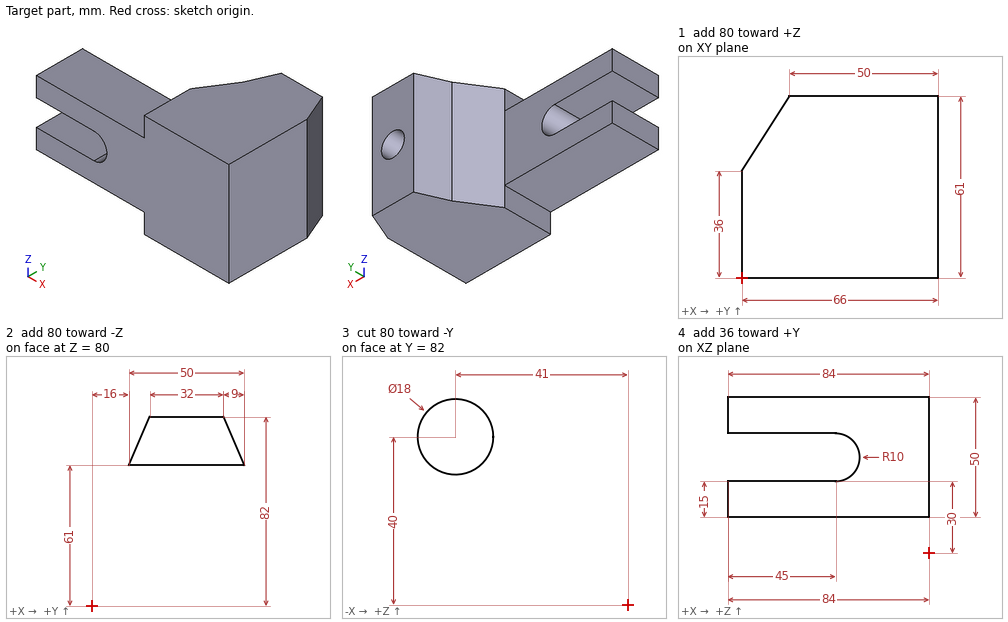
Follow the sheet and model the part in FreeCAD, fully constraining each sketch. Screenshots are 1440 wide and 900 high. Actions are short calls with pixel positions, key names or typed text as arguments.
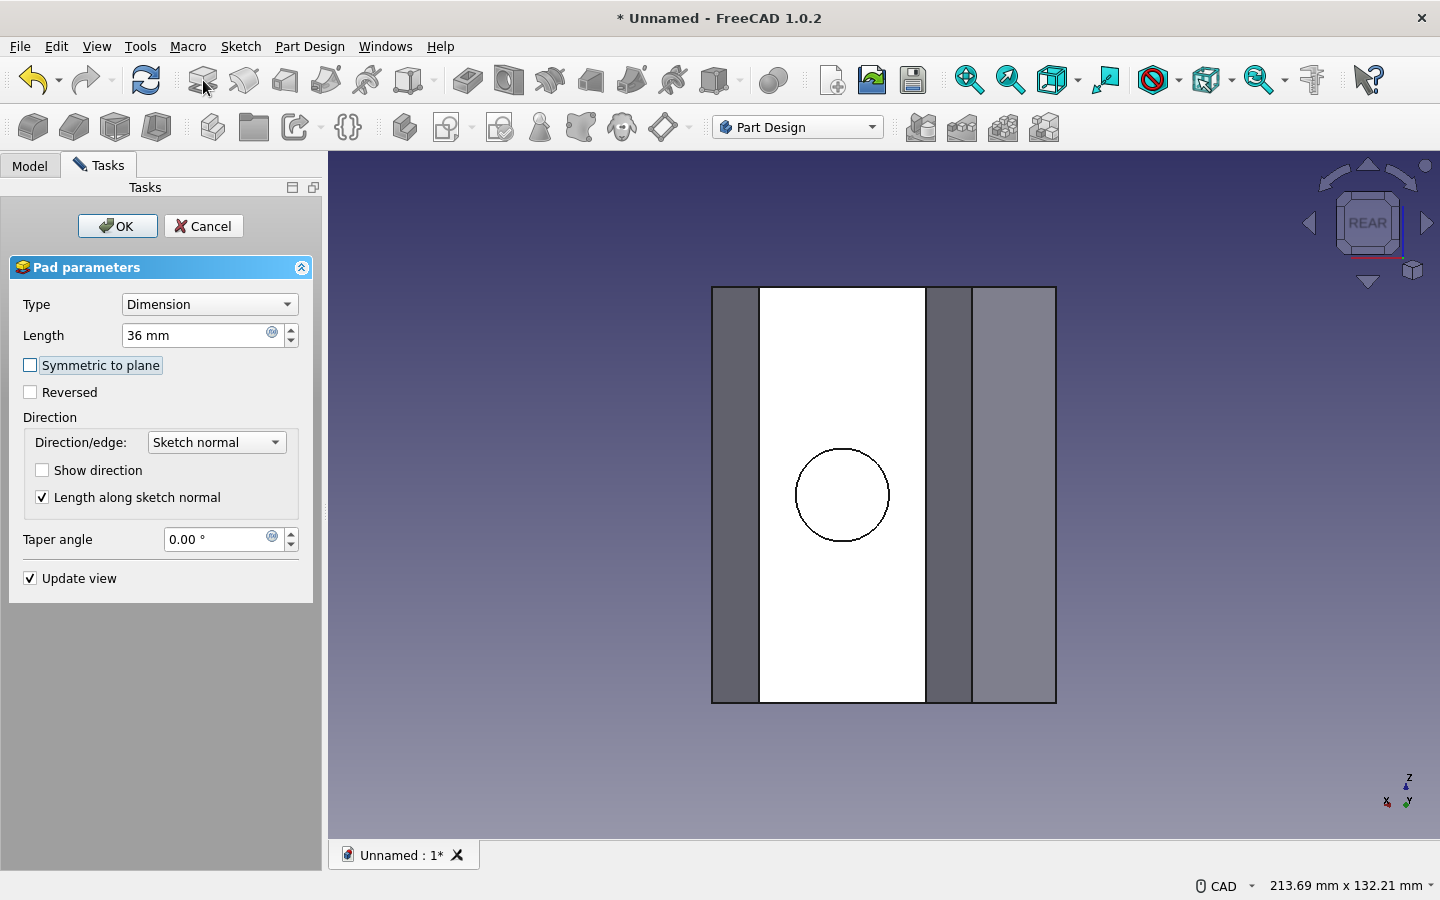
click(31, 392)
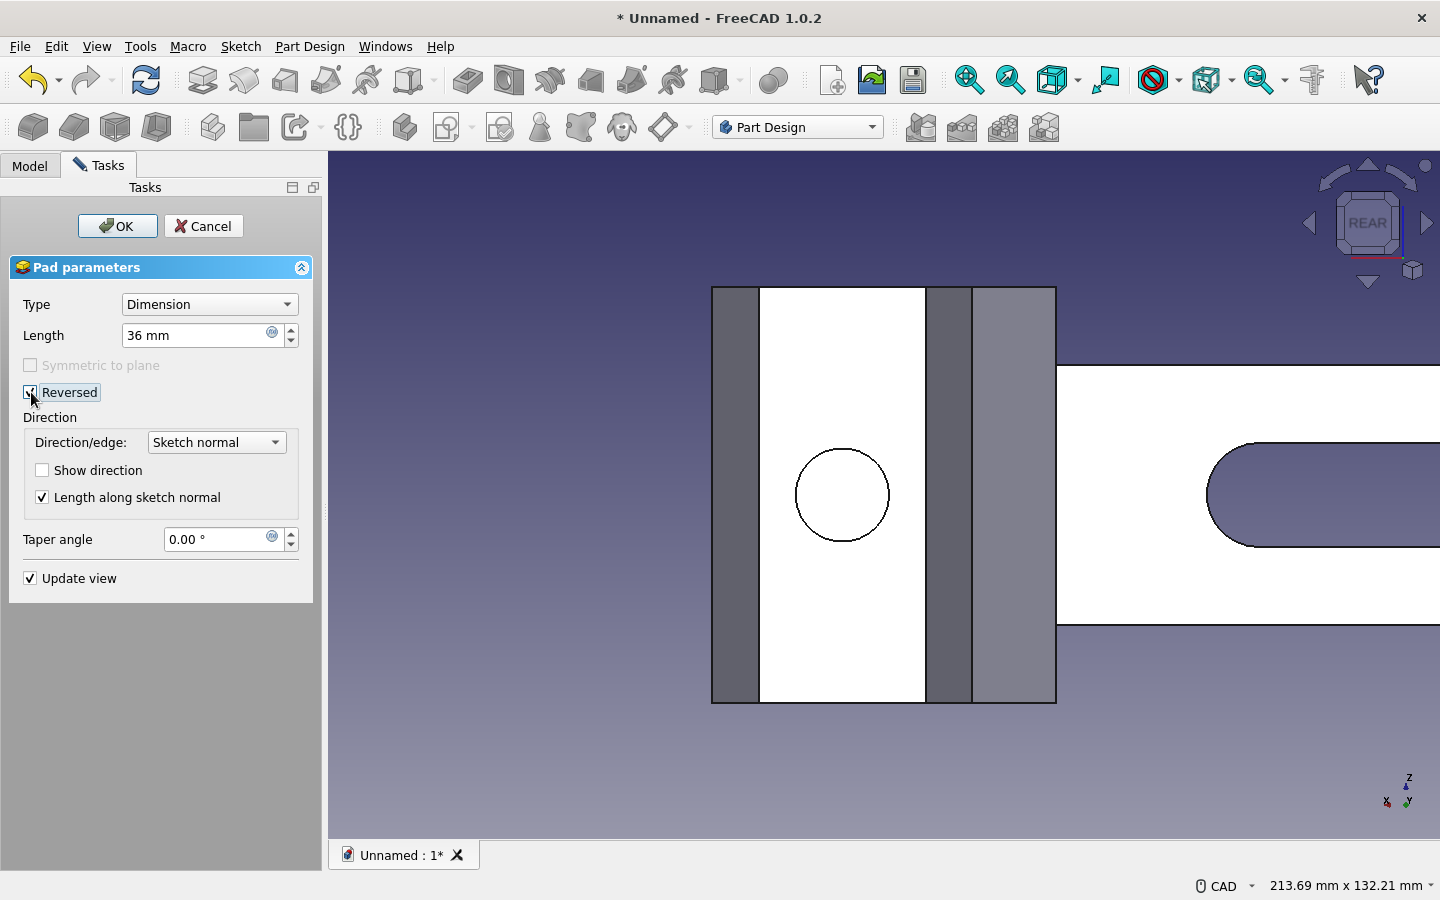
click(118, 226)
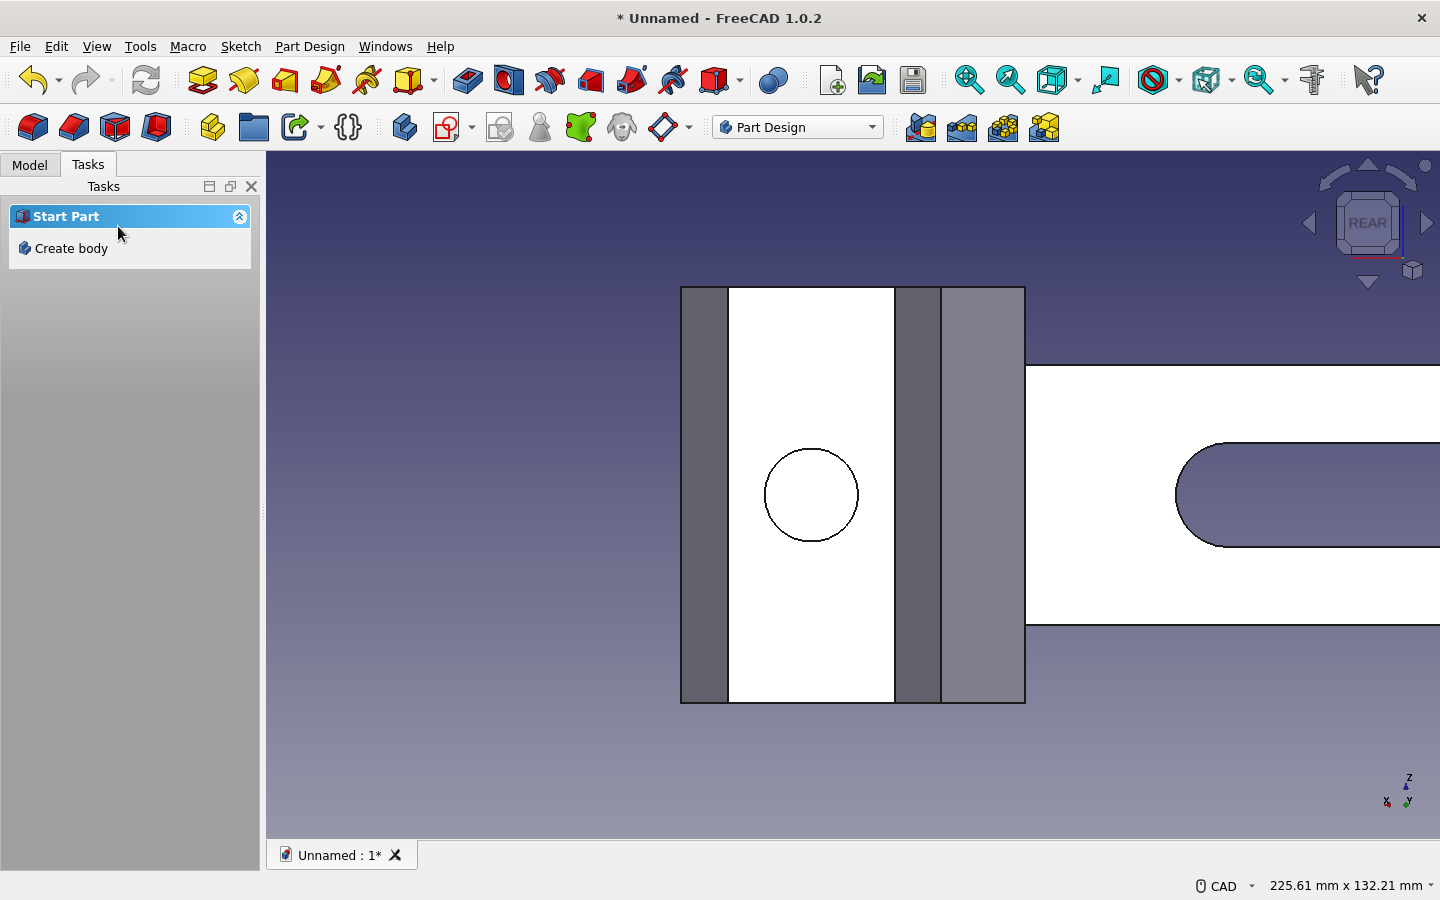
key(0)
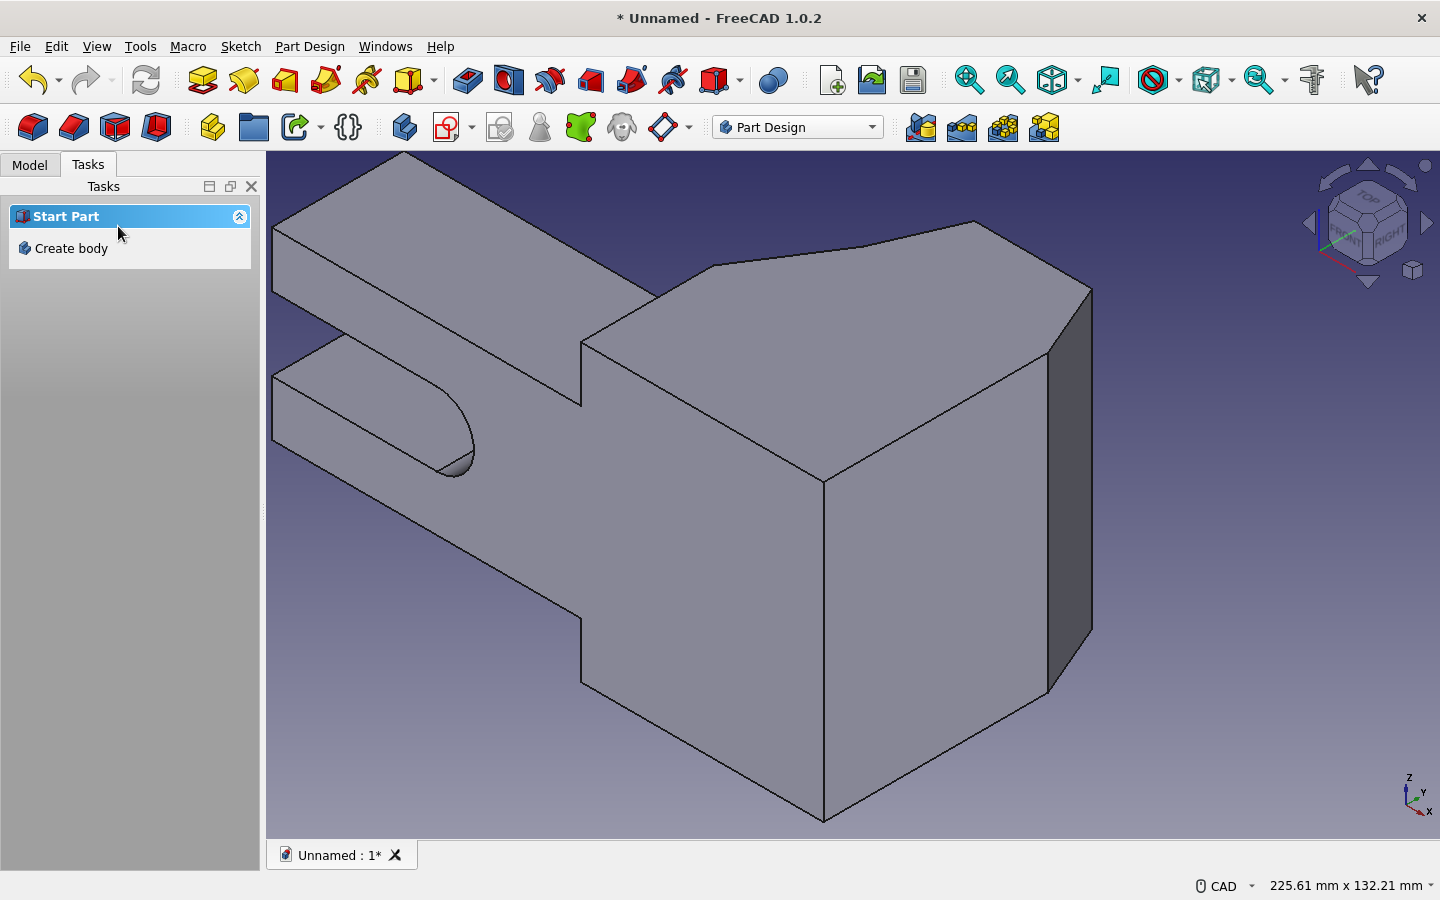
key(v)
key(f)